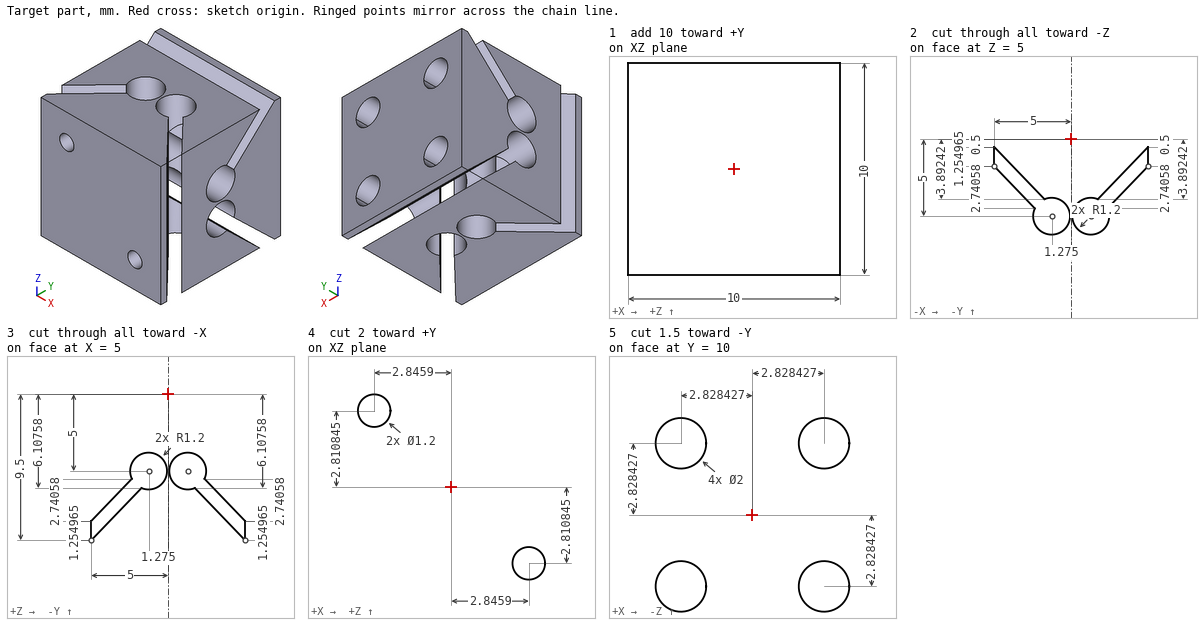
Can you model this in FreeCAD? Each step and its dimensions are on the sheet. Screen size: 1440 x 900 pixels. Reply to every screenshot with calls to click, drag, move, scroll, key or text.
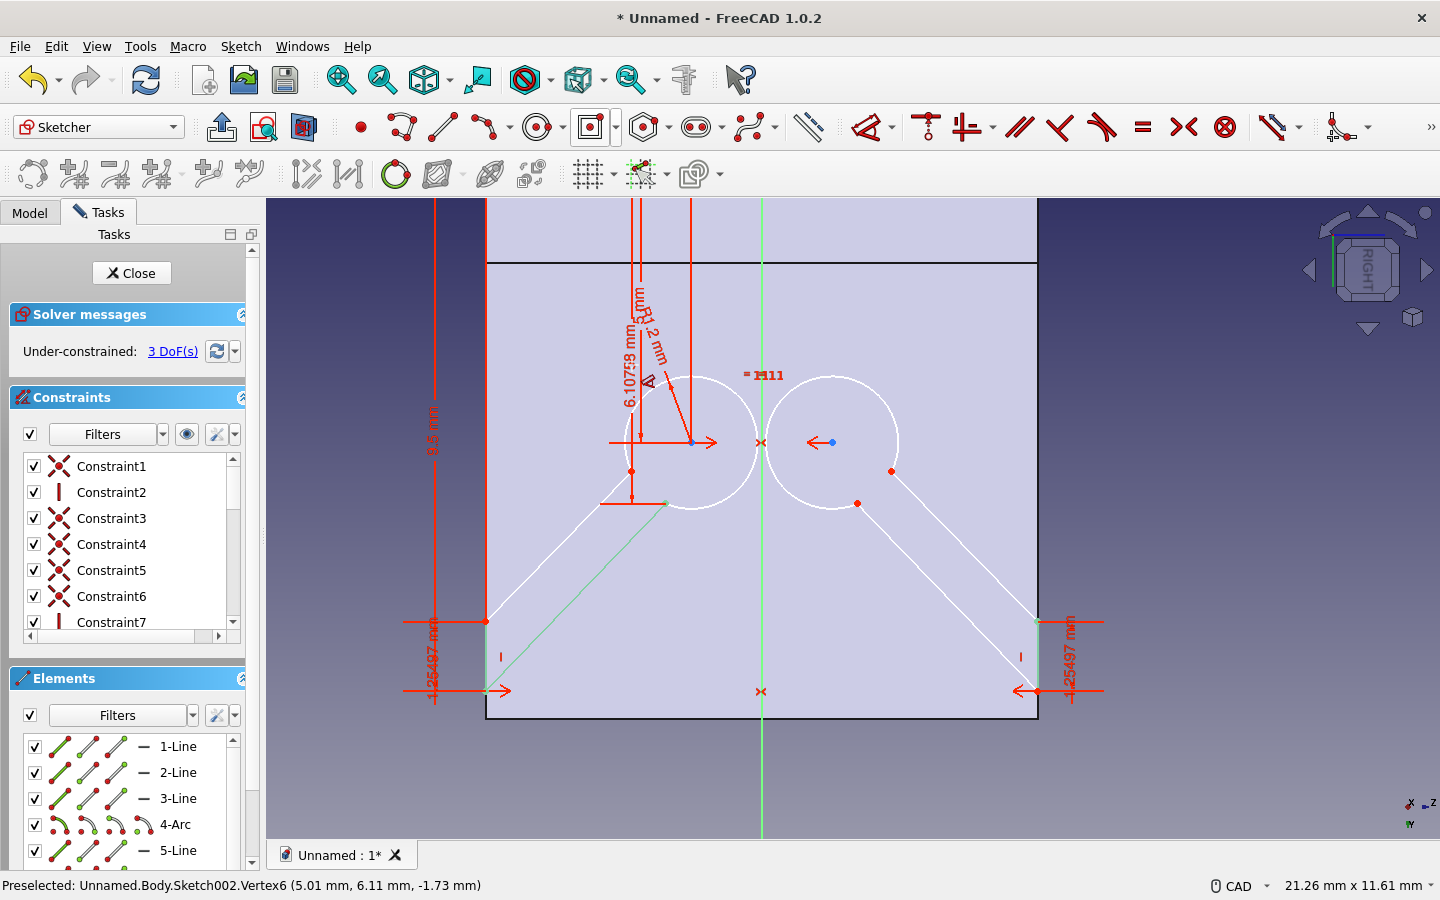
click(857, 504)
click(891, 365)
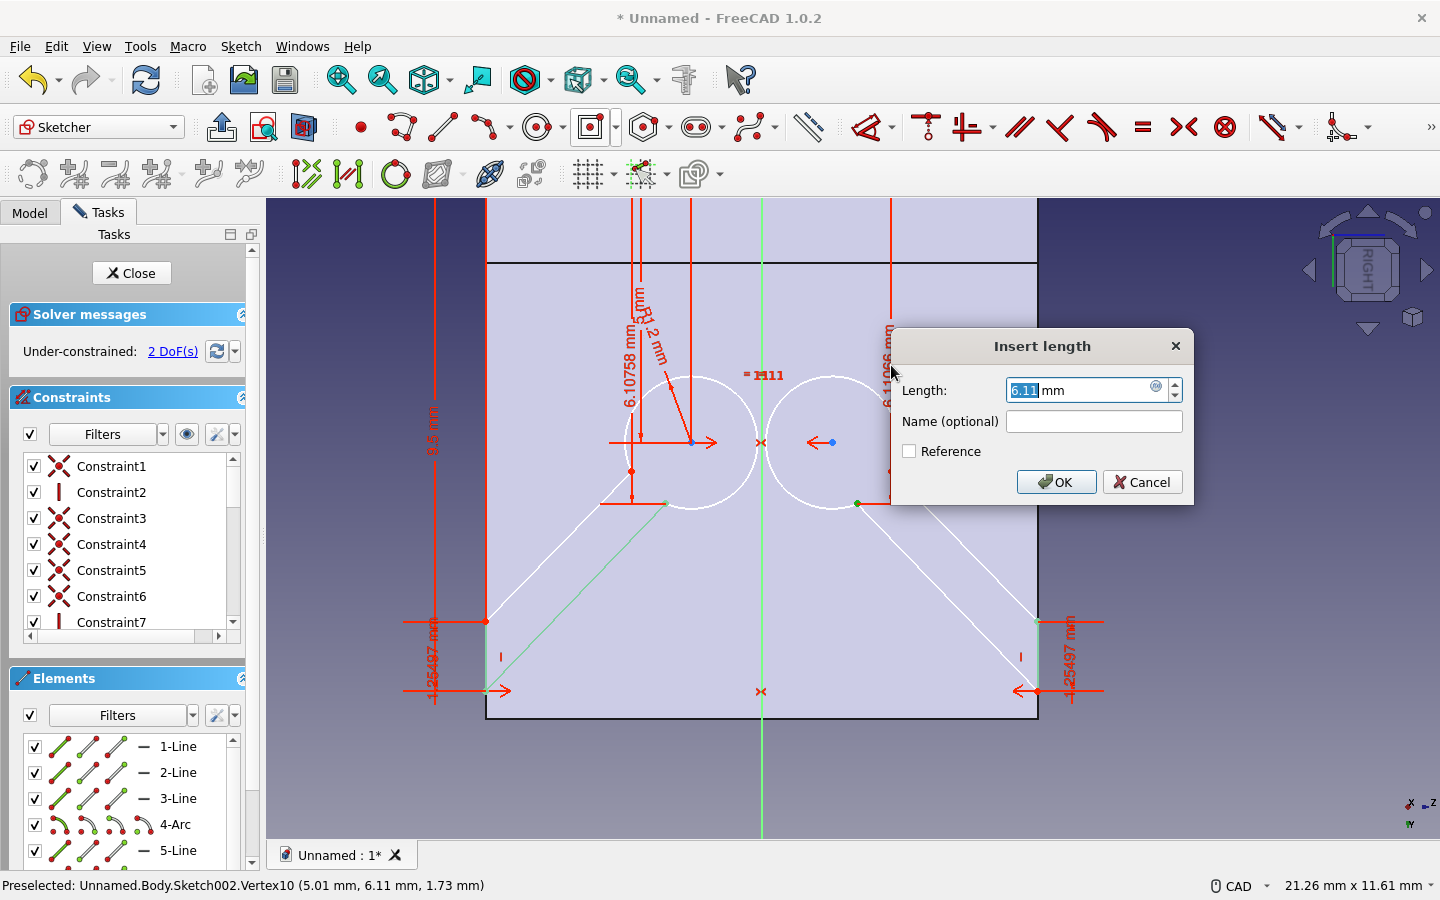
text(6.10758)
key(Return)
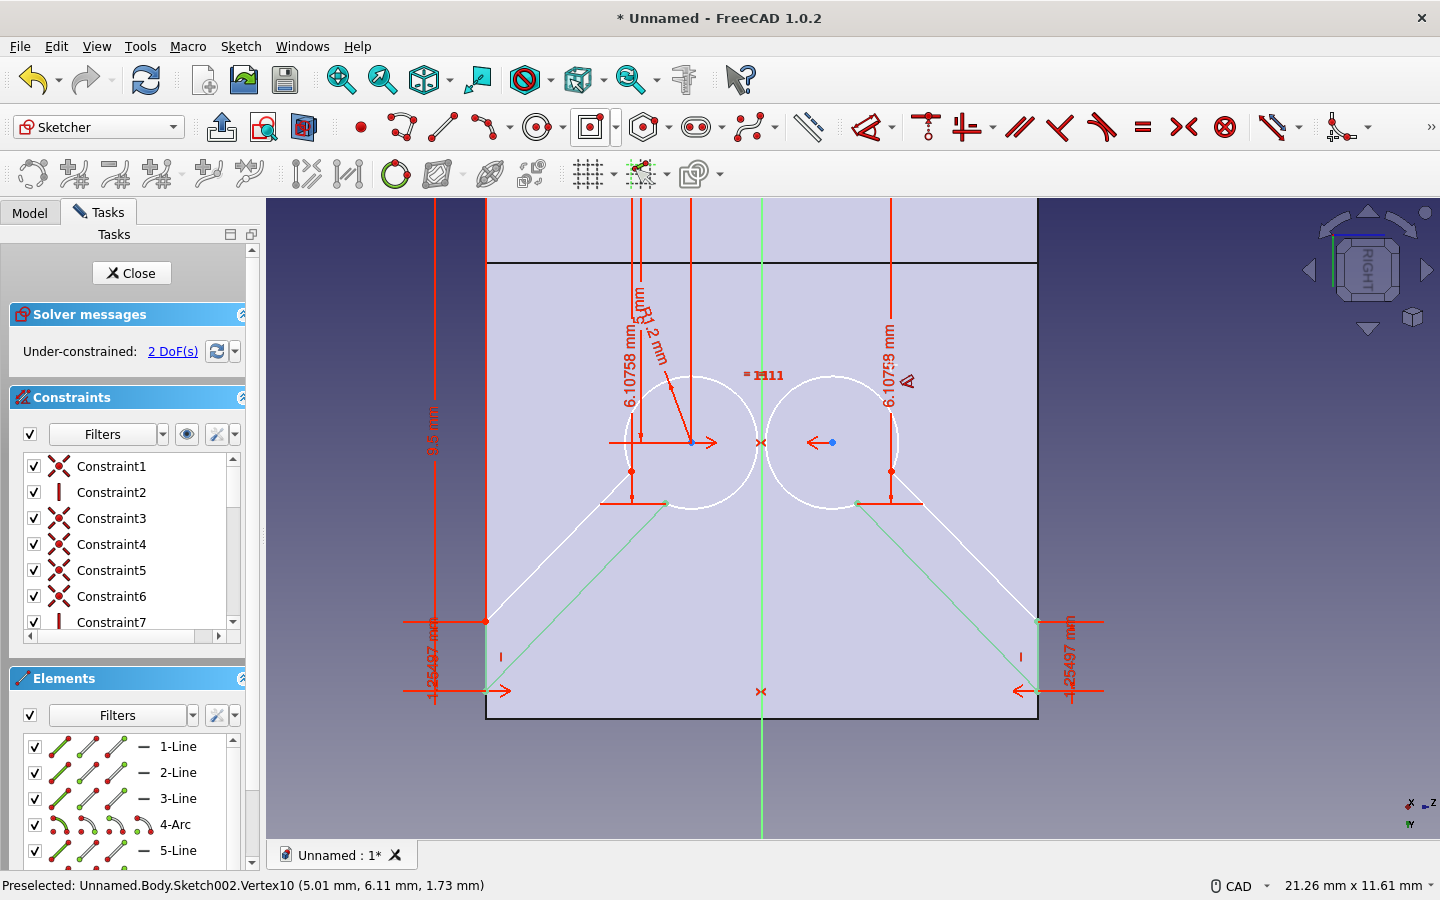
click(588, 517)
click(452, 547)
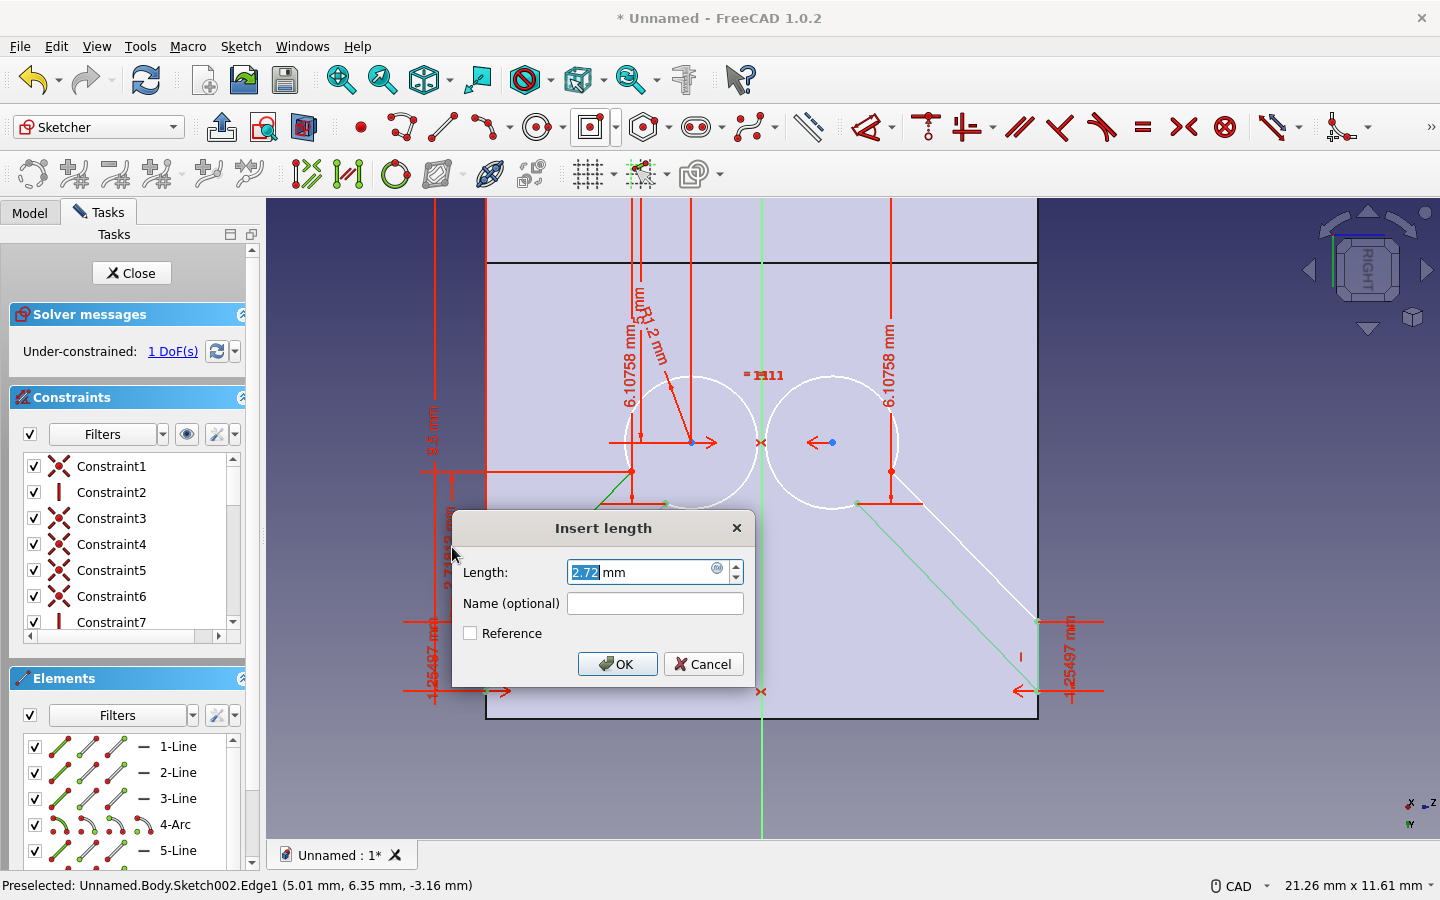
text(2.74058)
key(Return)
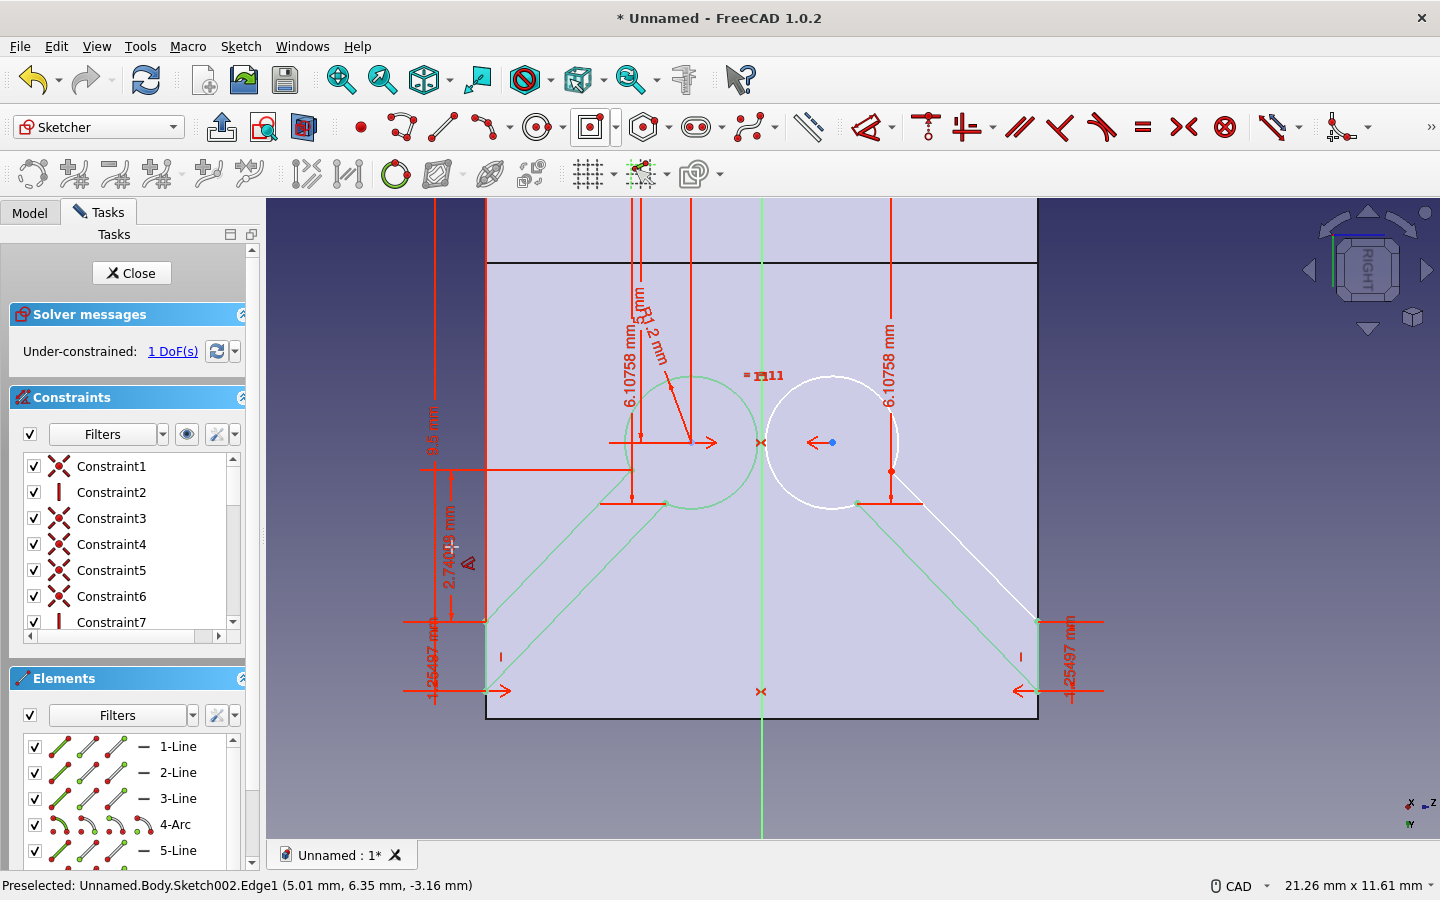
click(994, 577)
click(1072, 547)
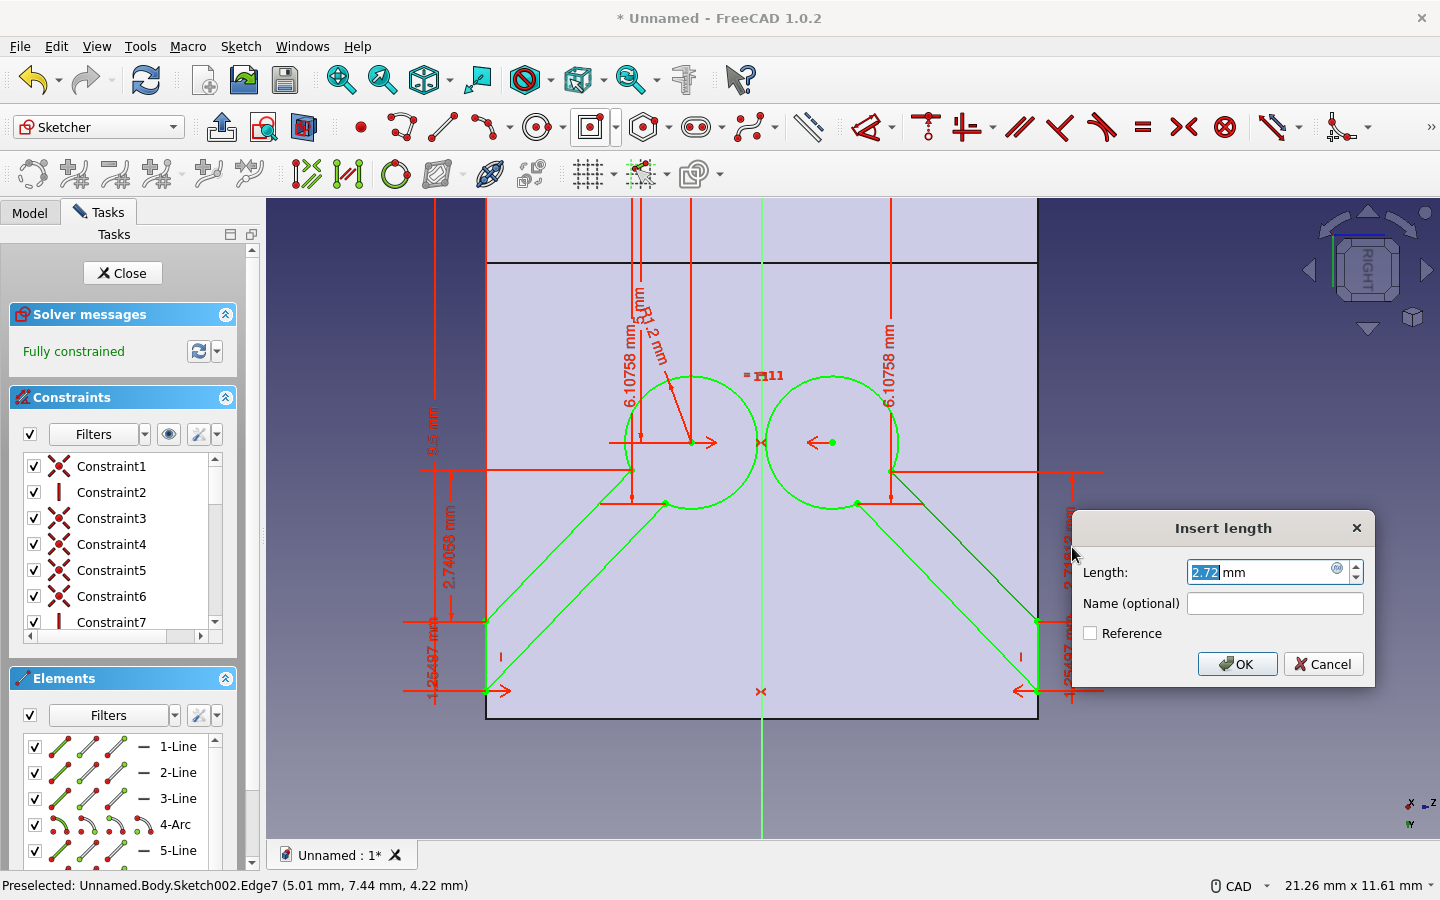
text(2.74058)
key(Return)
key(Escape)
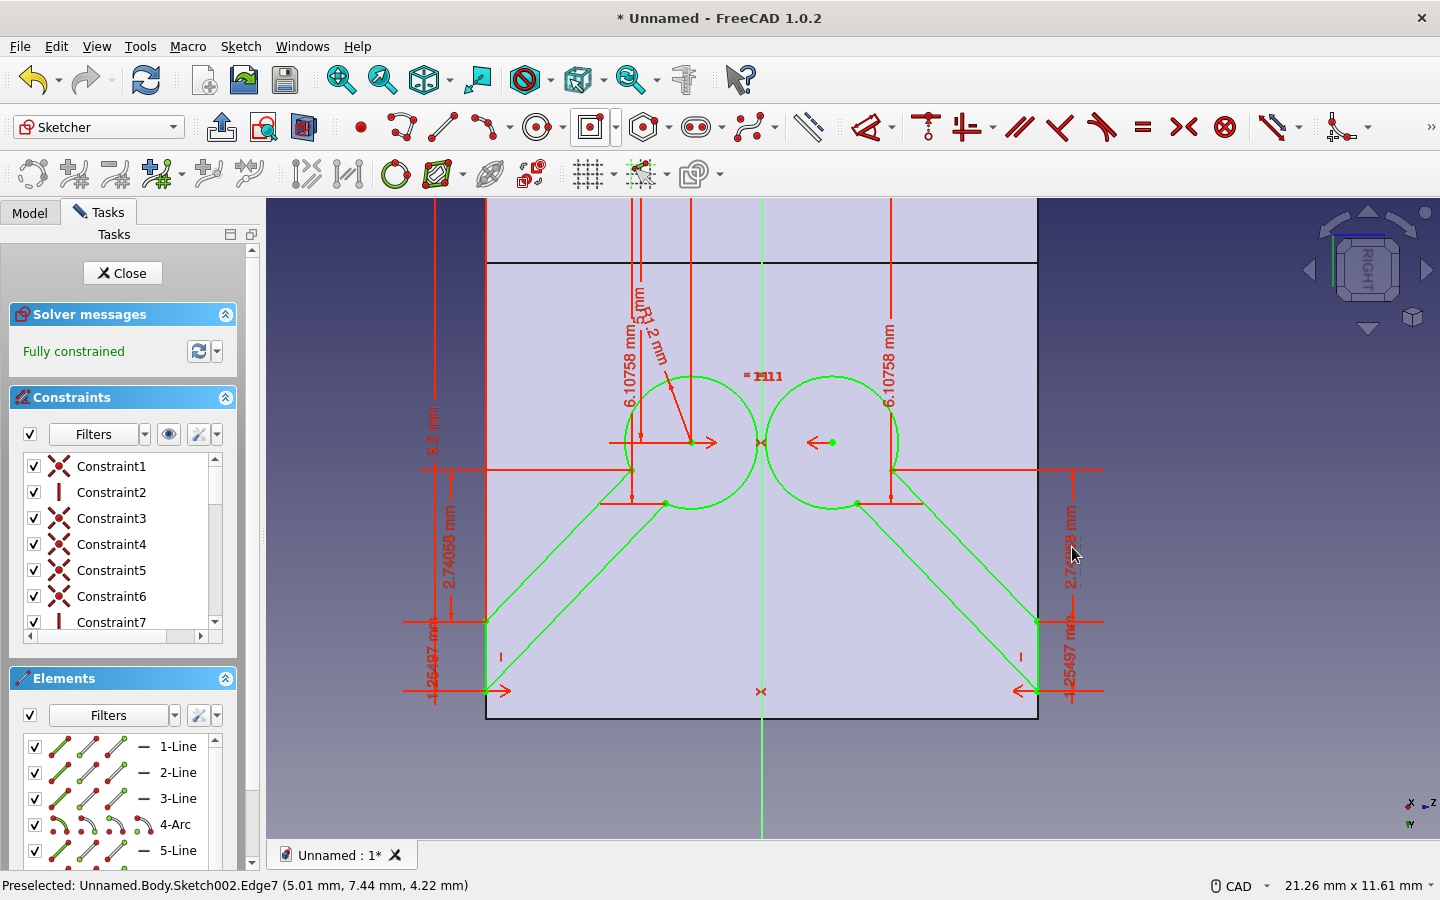
click(123, 273)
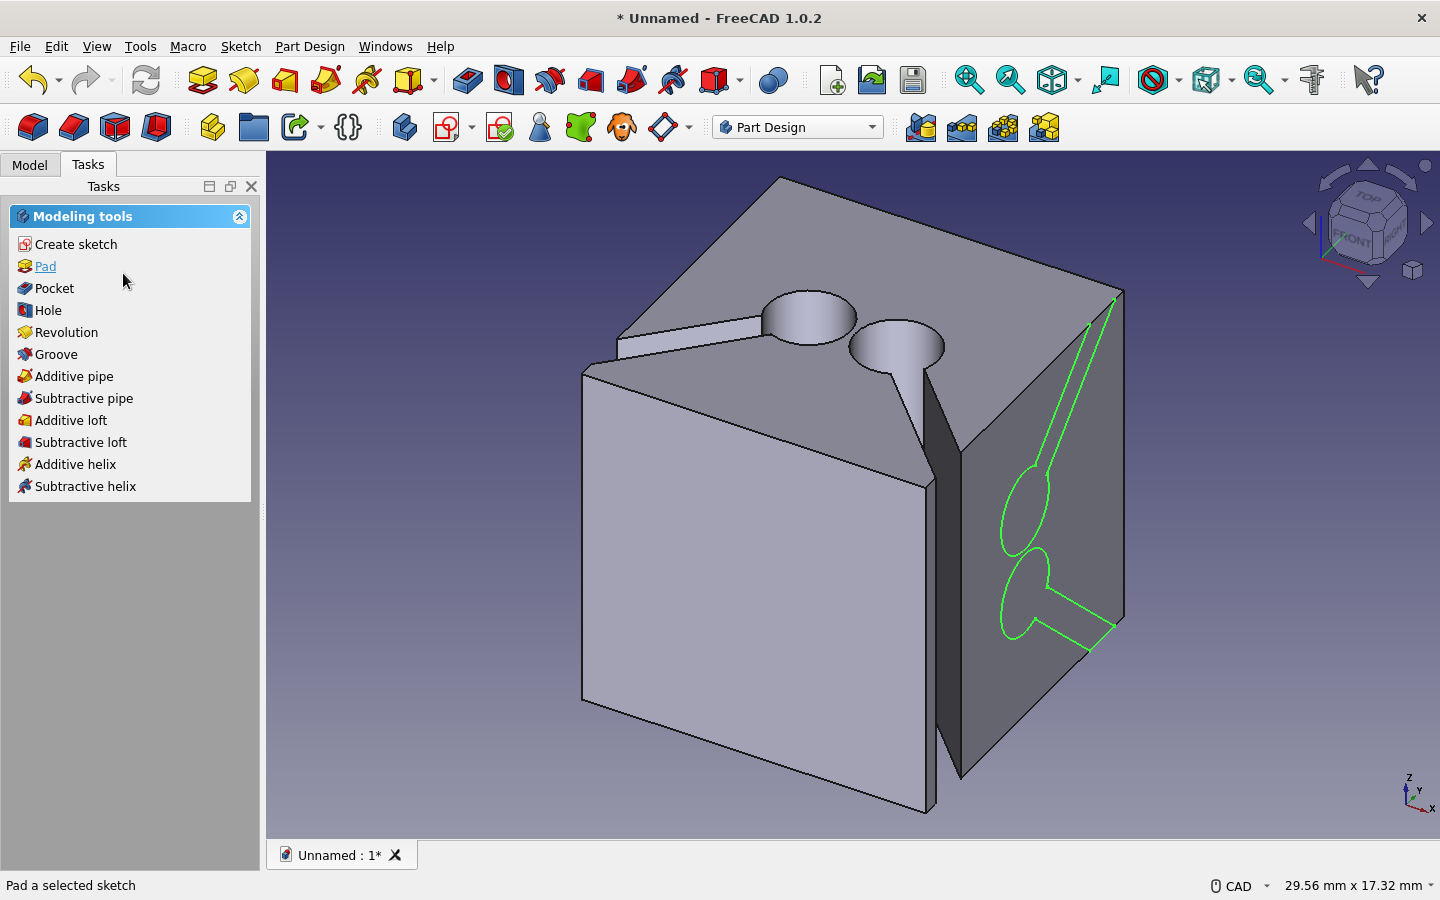
click(468, 80)